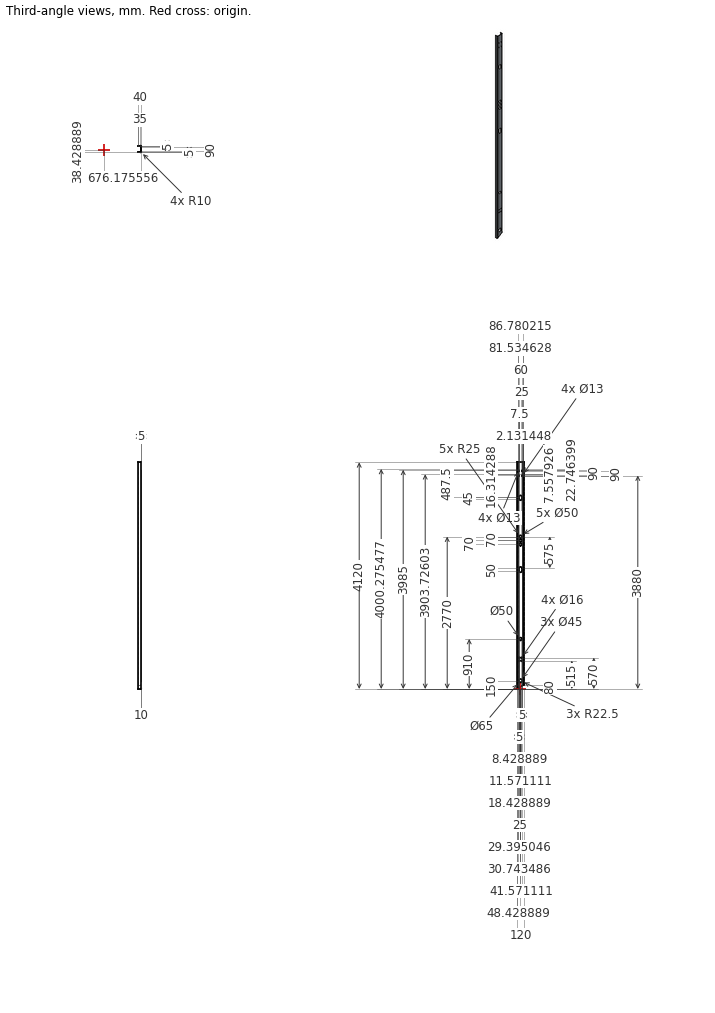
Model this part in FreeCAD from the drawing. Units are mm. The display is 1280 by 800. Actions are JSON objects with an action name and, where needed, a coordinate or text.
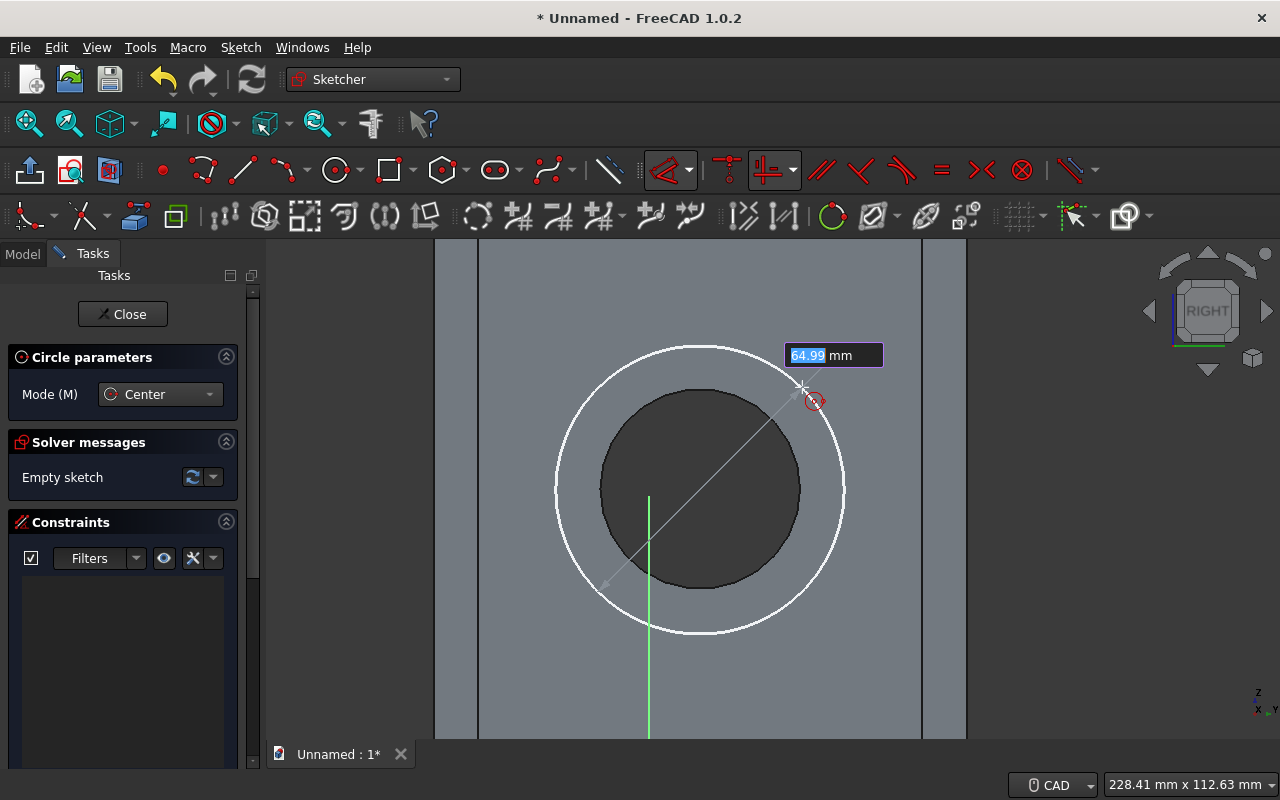
{"action": "type", "text": "65"}
{"action": "key", "text": "Return"}
{"action": "key", "text": "Escape"}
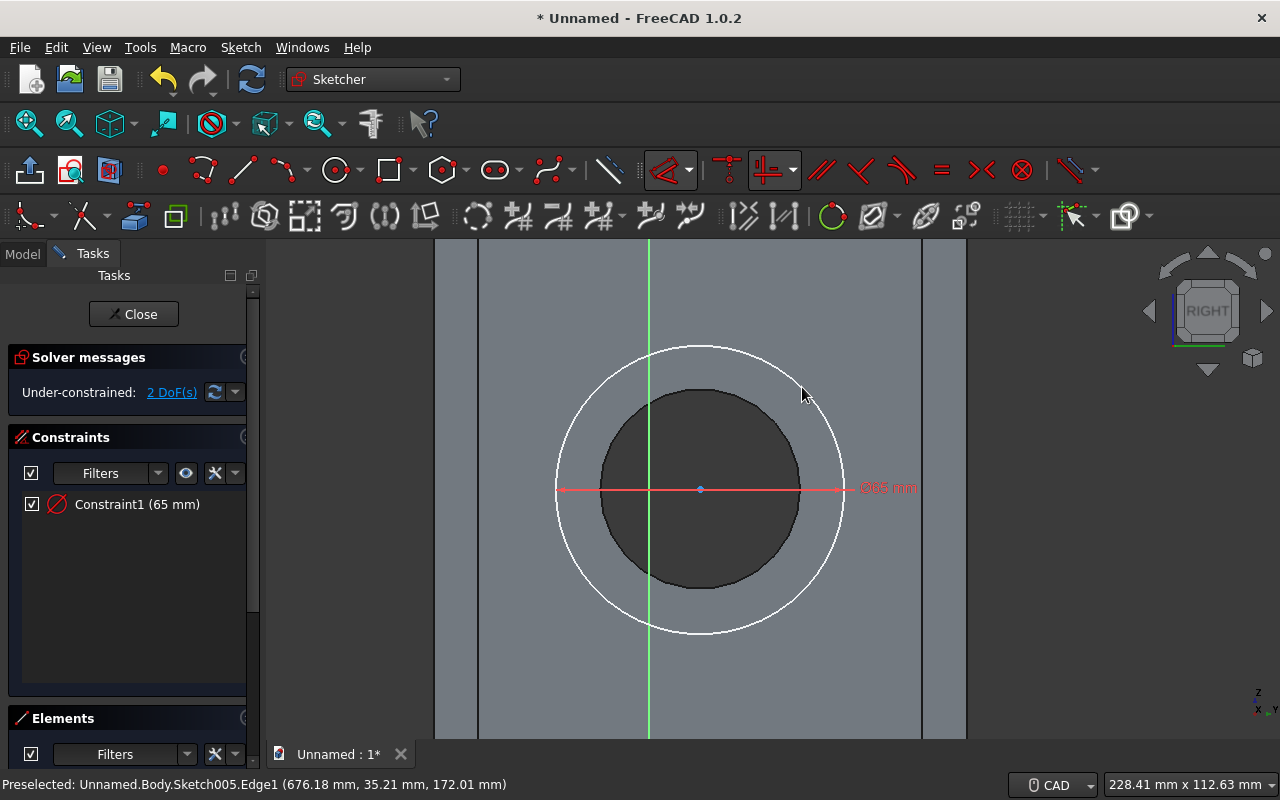
{"action": "left_click", "coordinate": [700, 490]}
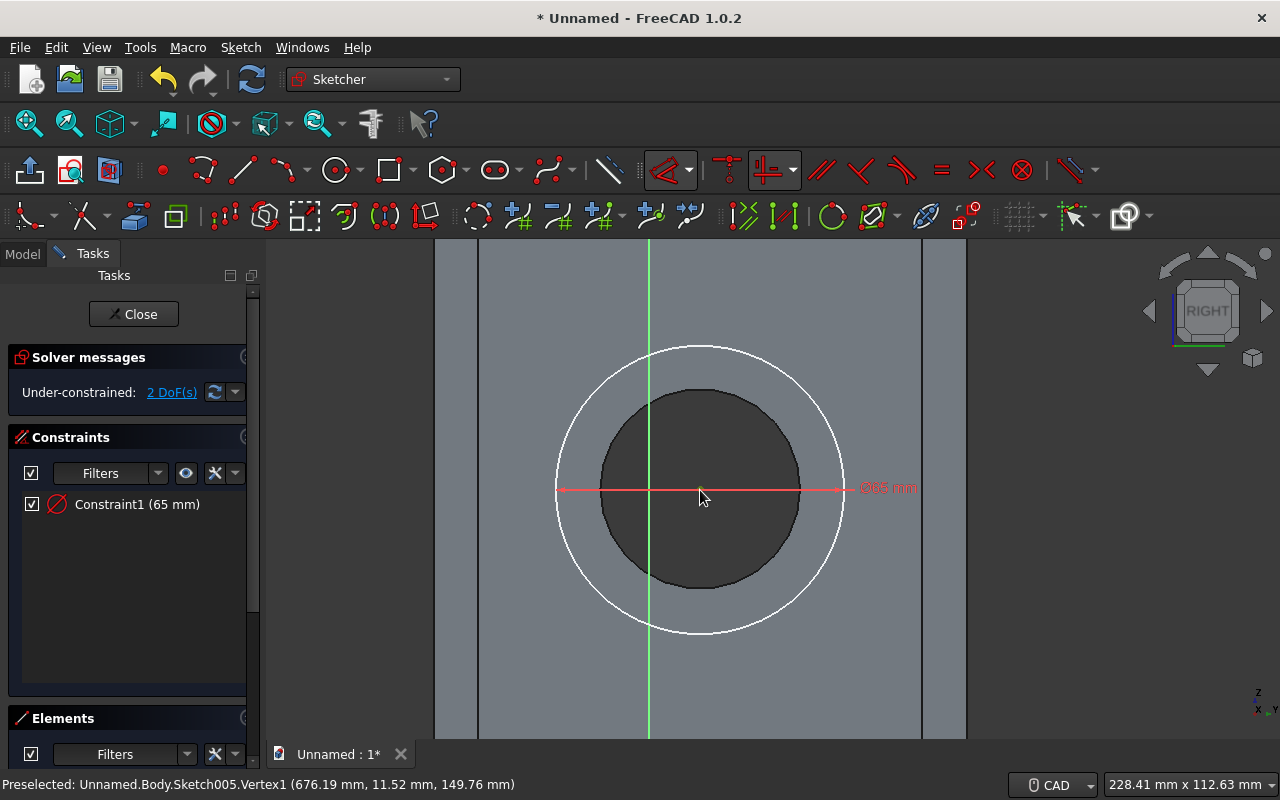
{"action": "key", "text": "i"}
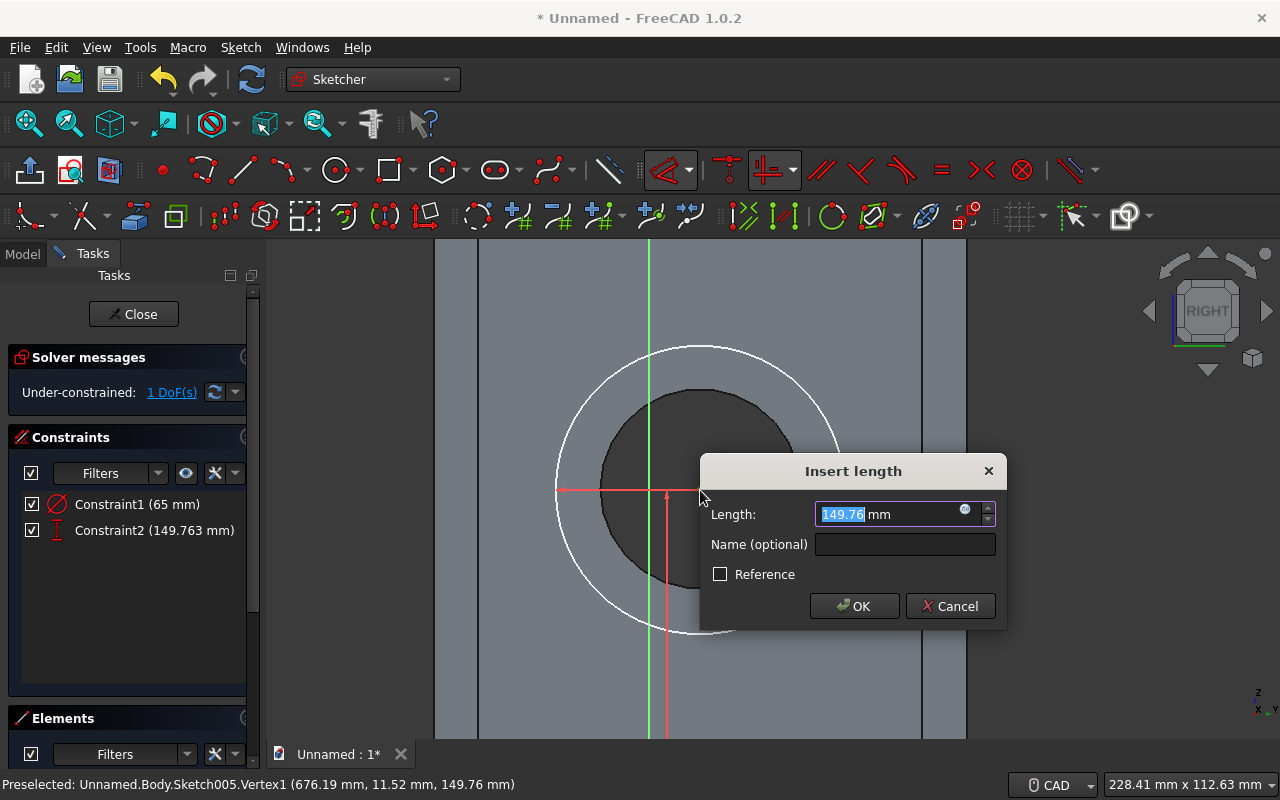
{"action": "type", "text": "150"}
{"action": "key", "text": "Return"}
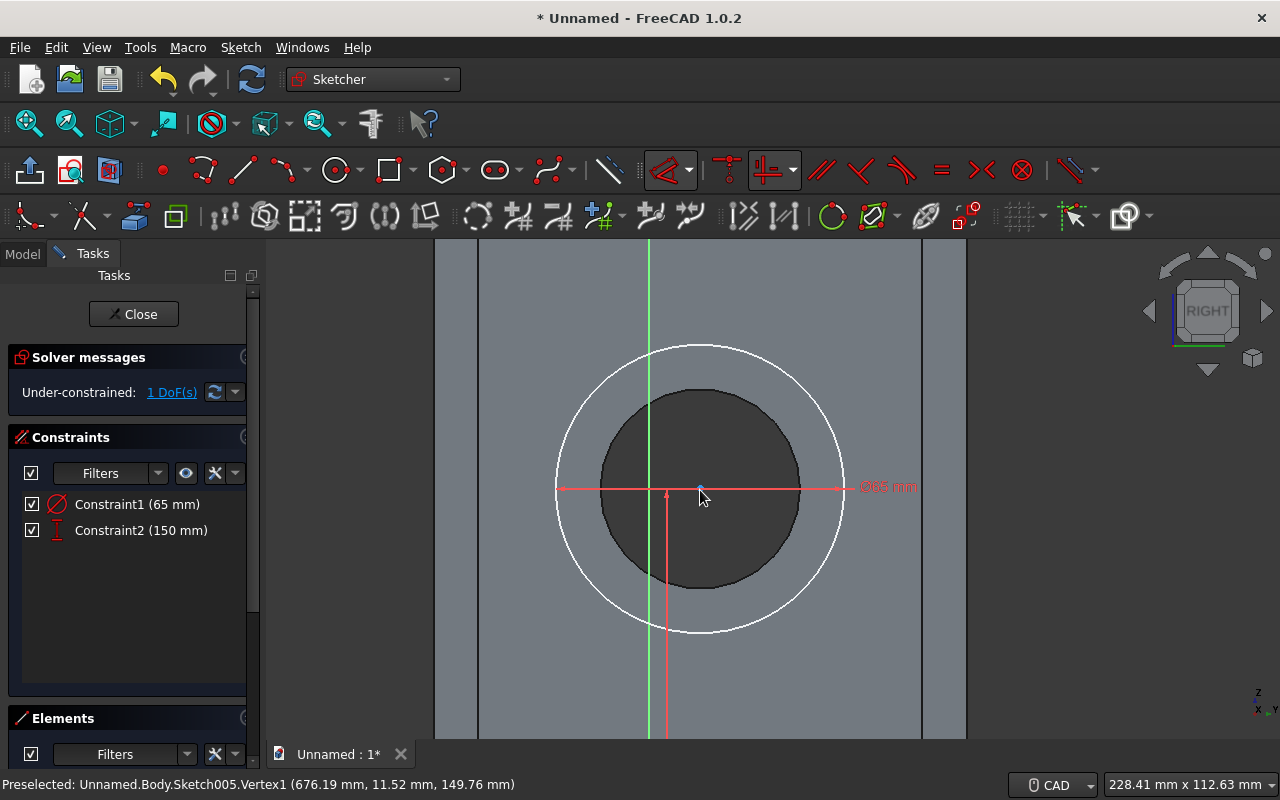
{"action": "left_click", "coordinate": [700, 489]}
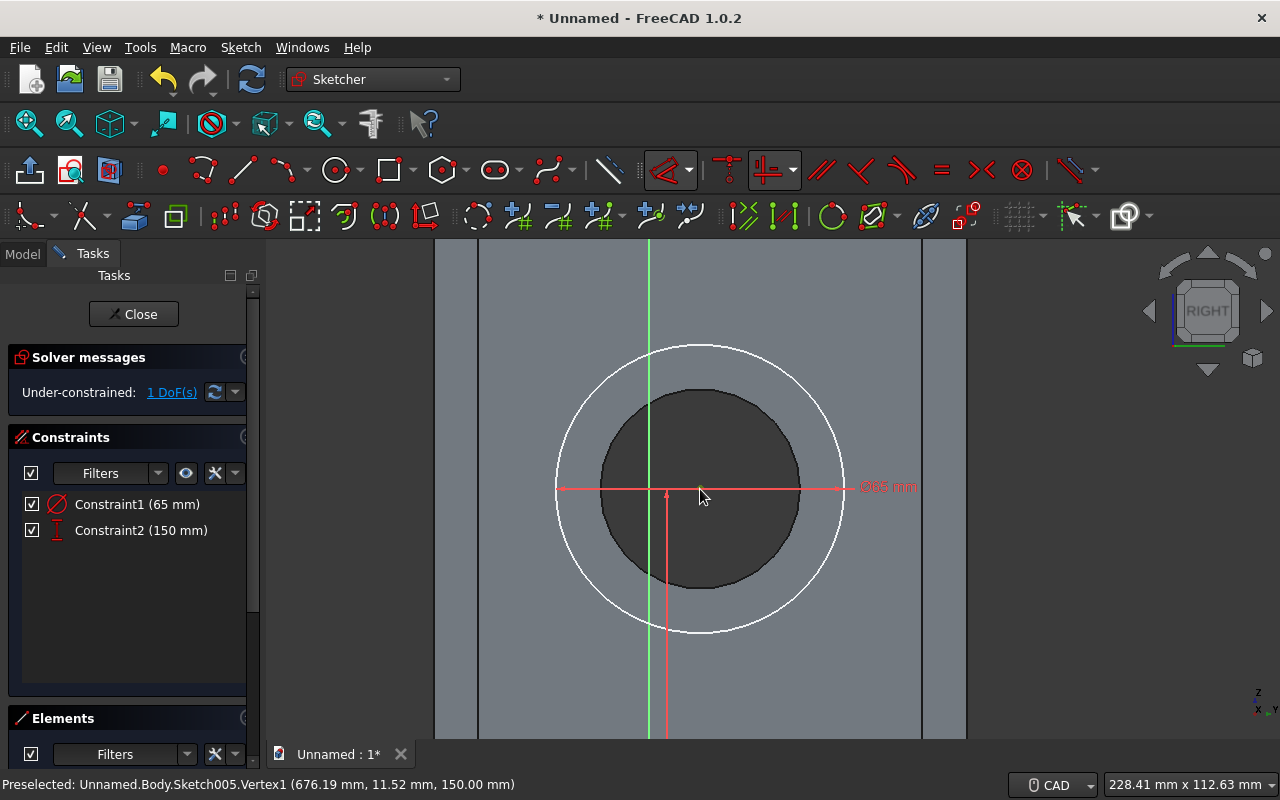
{"action": "key", "text": "l"}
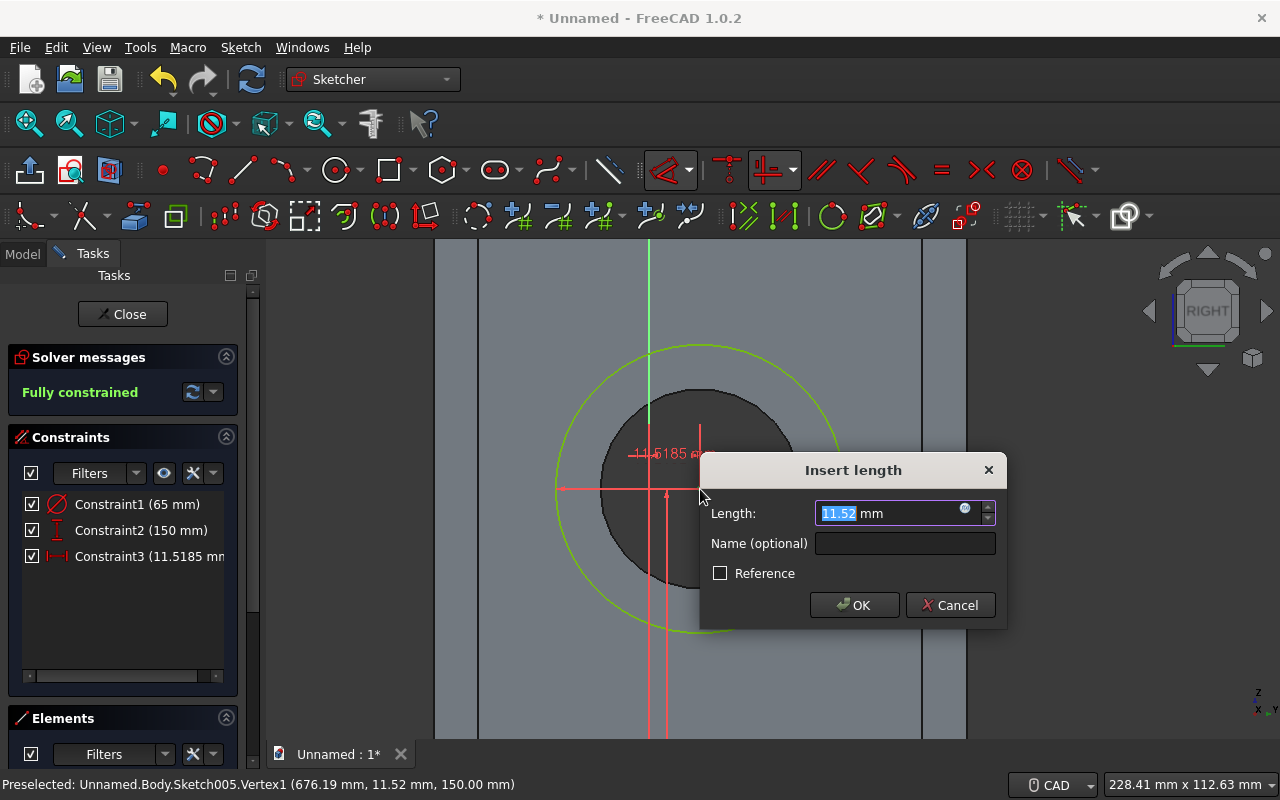
{"action": "type", "text": "11.571111"}
{"action": "key", "text": "Return"}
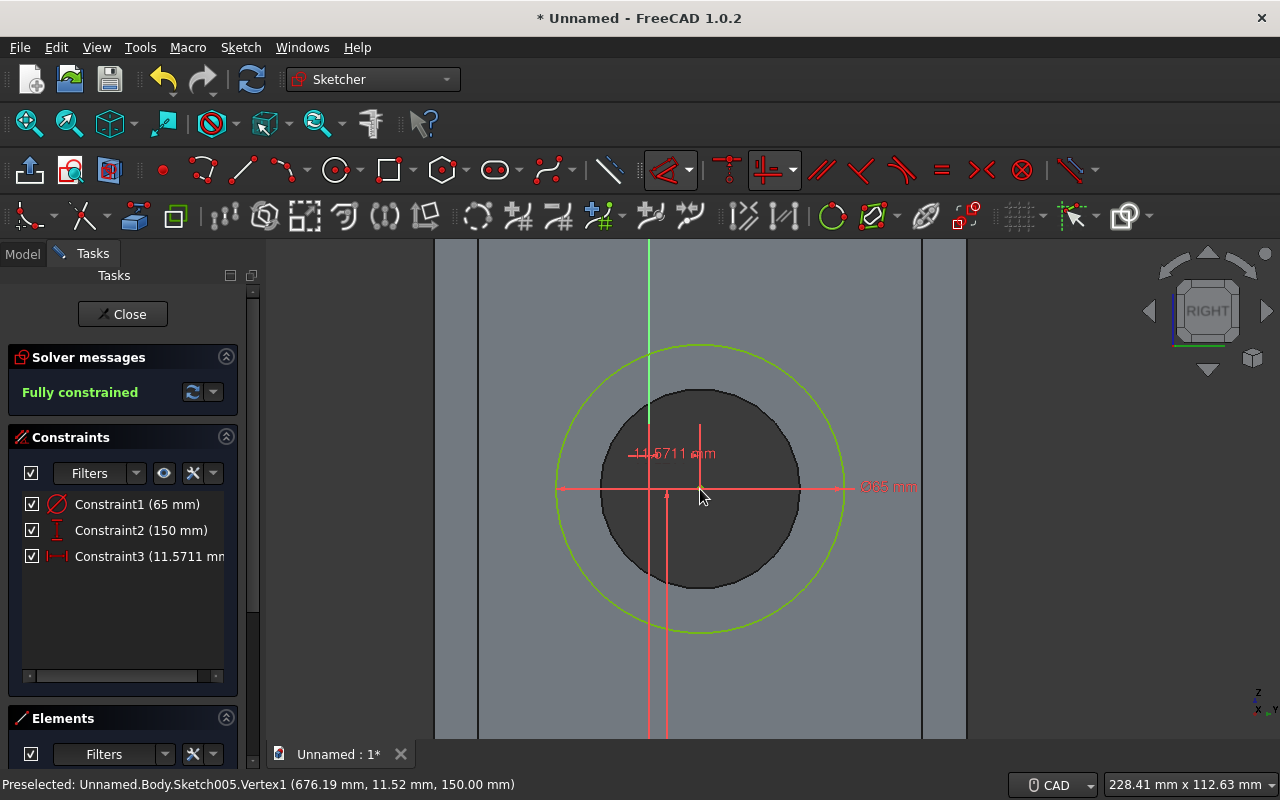
{"action": "left_click", "coordinate": [123, 314]}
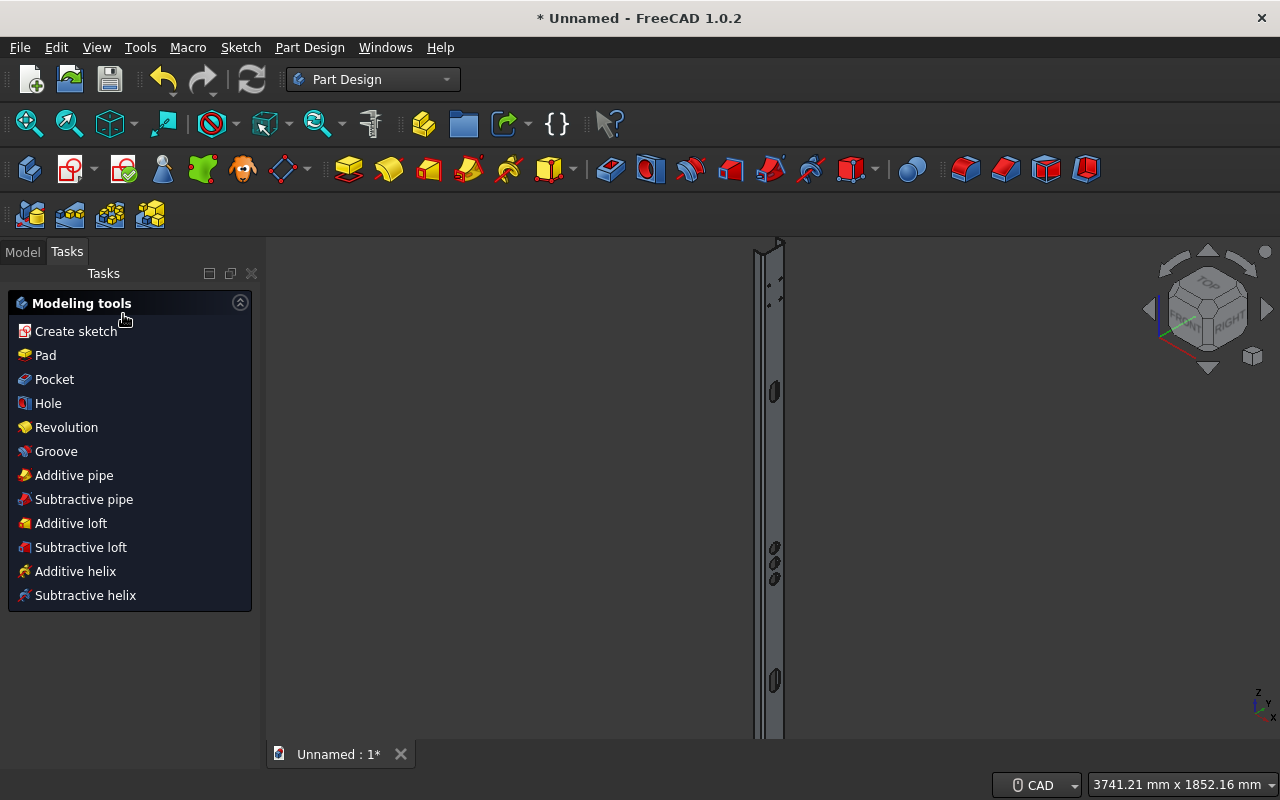
{"action": "left_click", "coordinate": [612, 170]}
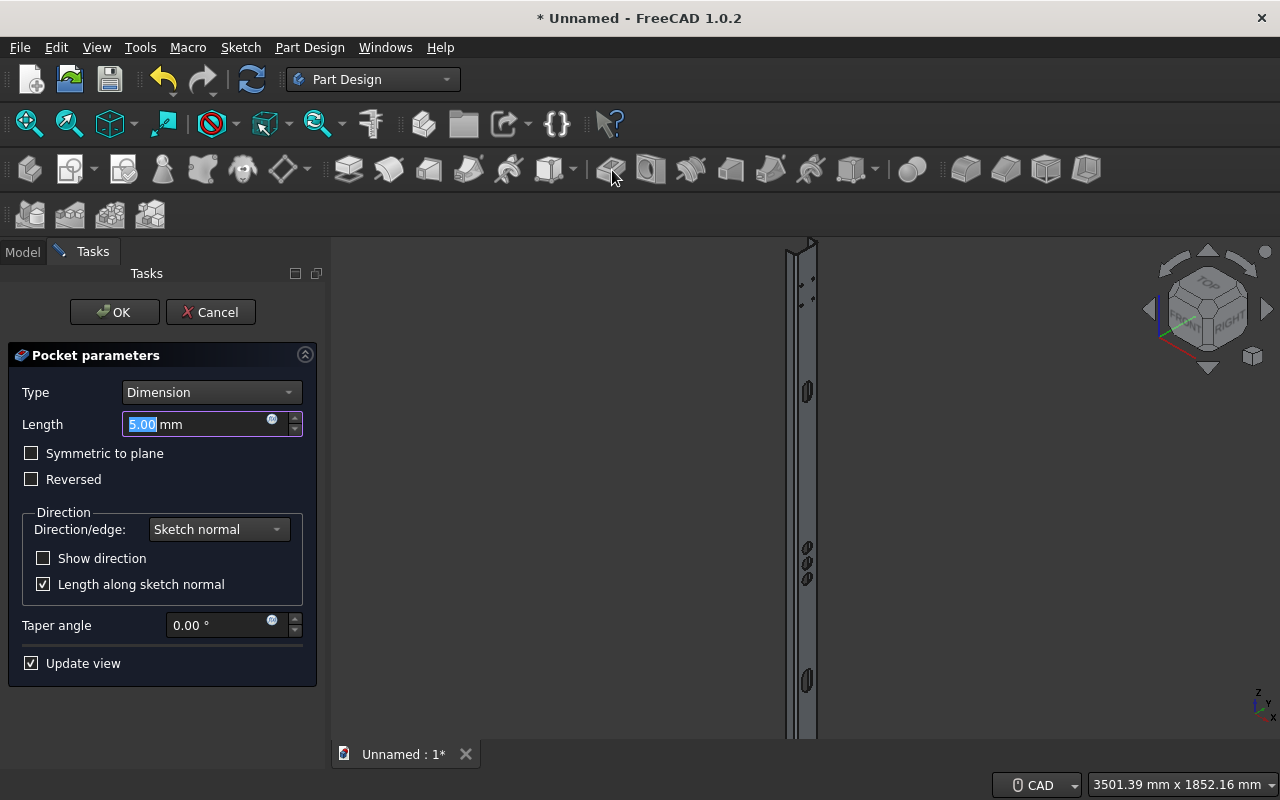
{"action": "type", "text": "10"}
{"action": "key", "text": "Tab"}